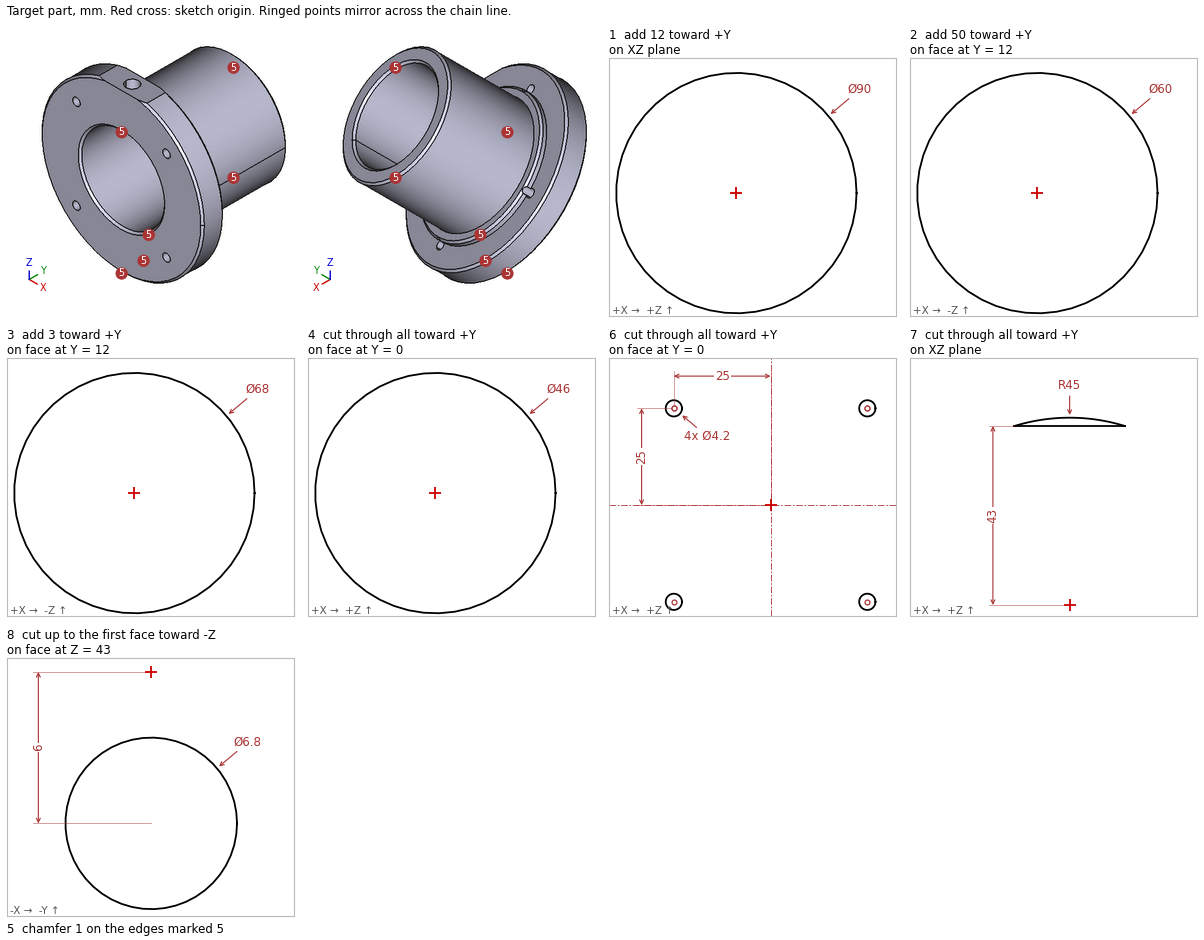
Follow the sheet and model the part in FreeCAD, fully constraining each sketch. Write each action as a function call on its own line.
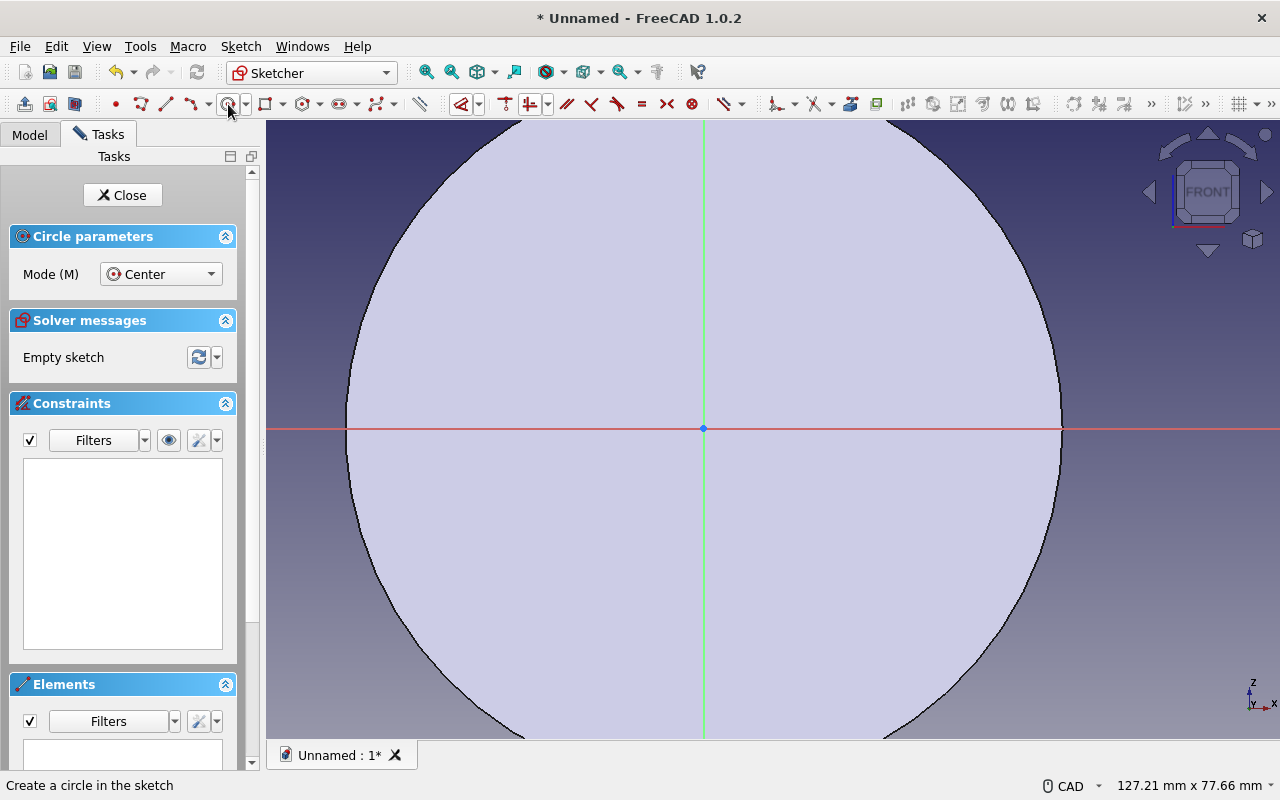
click(704, 429)
move(834, 299)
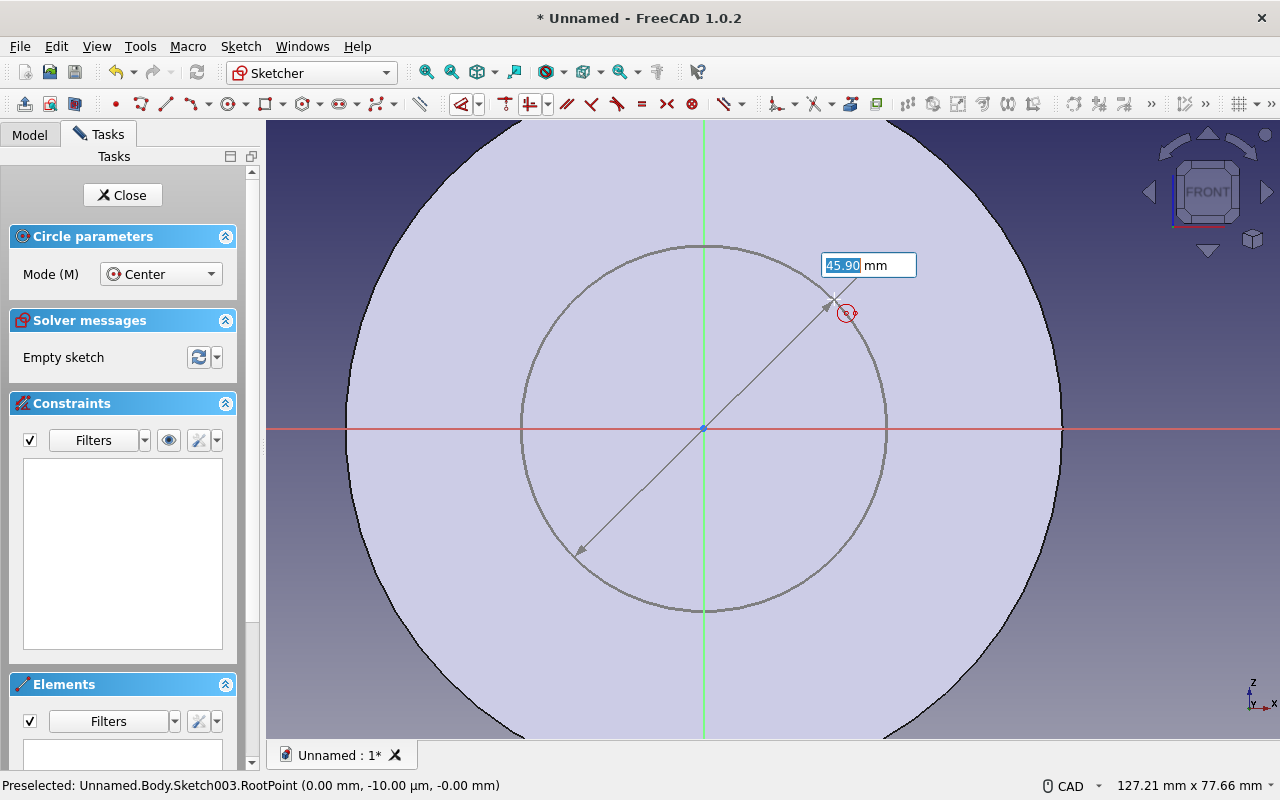
text(46)
key(Return)
key(Escape)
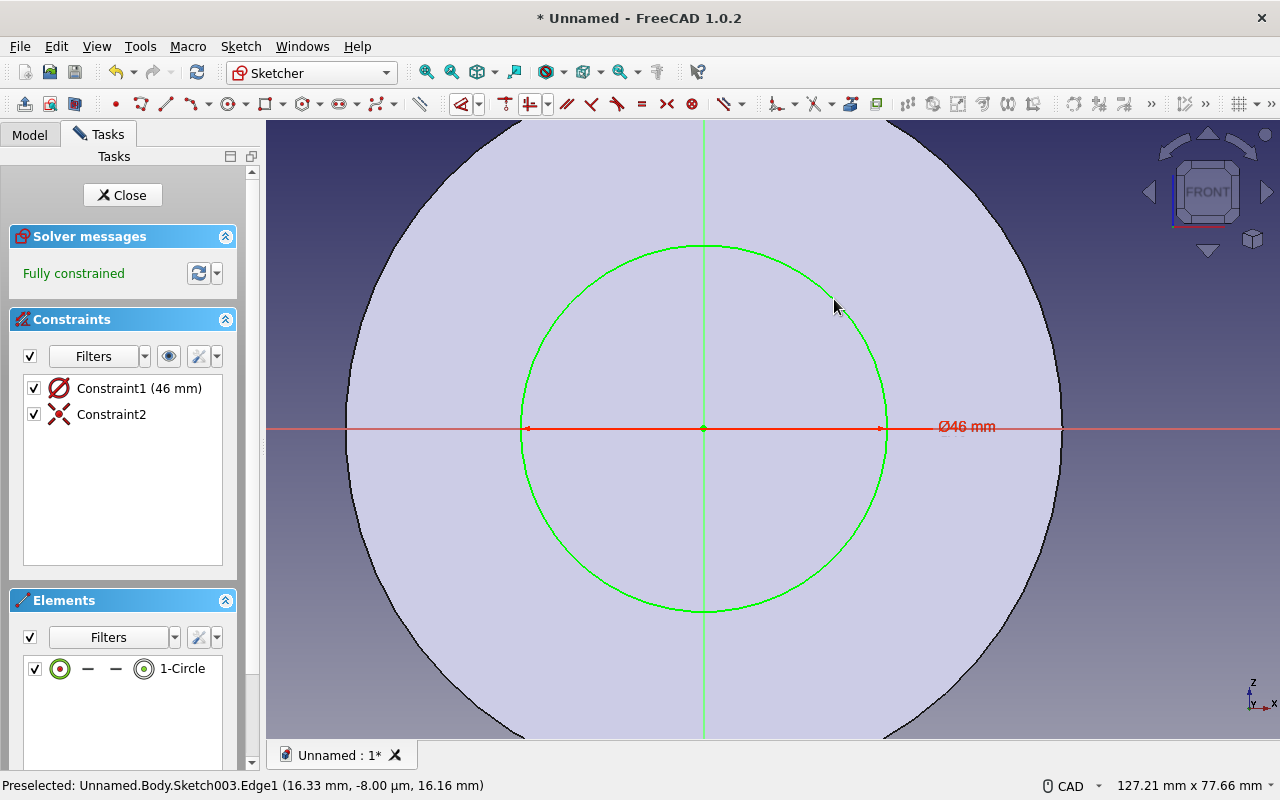
click(123, 195)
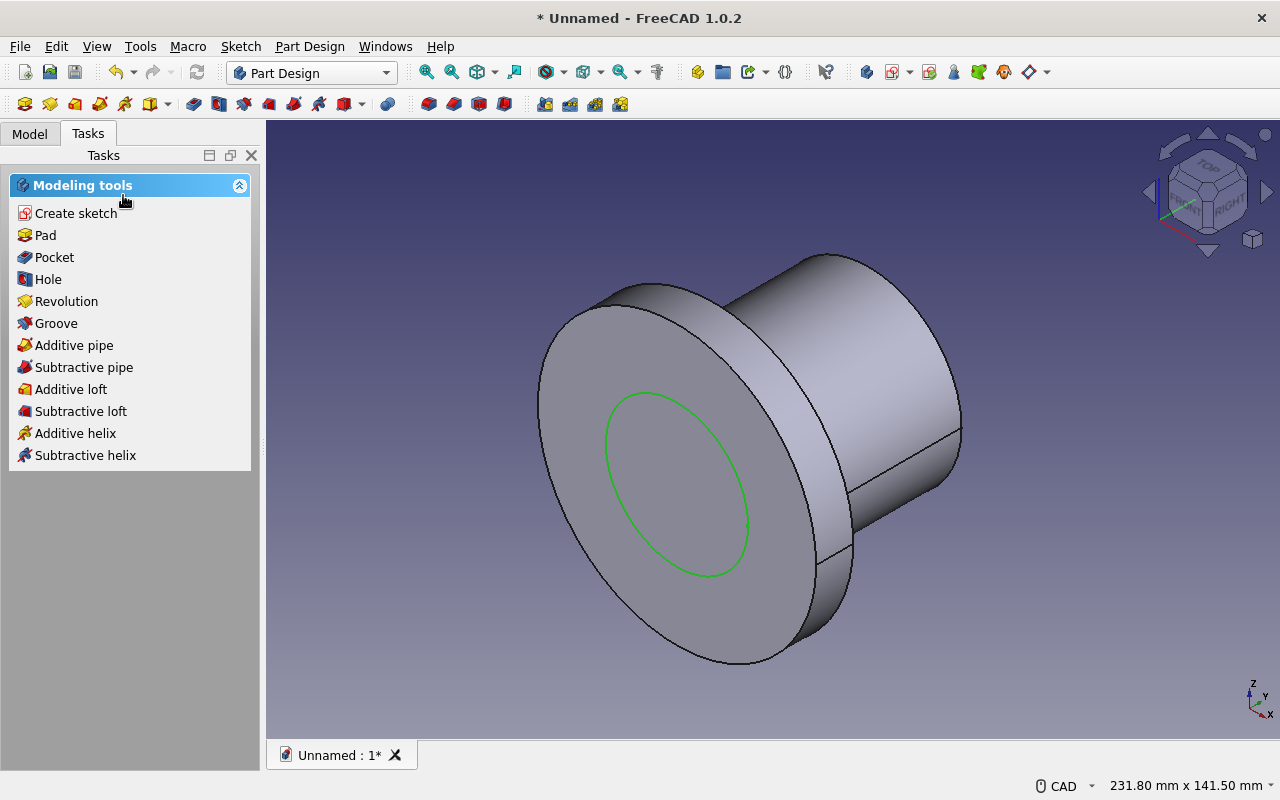
click(194, 104)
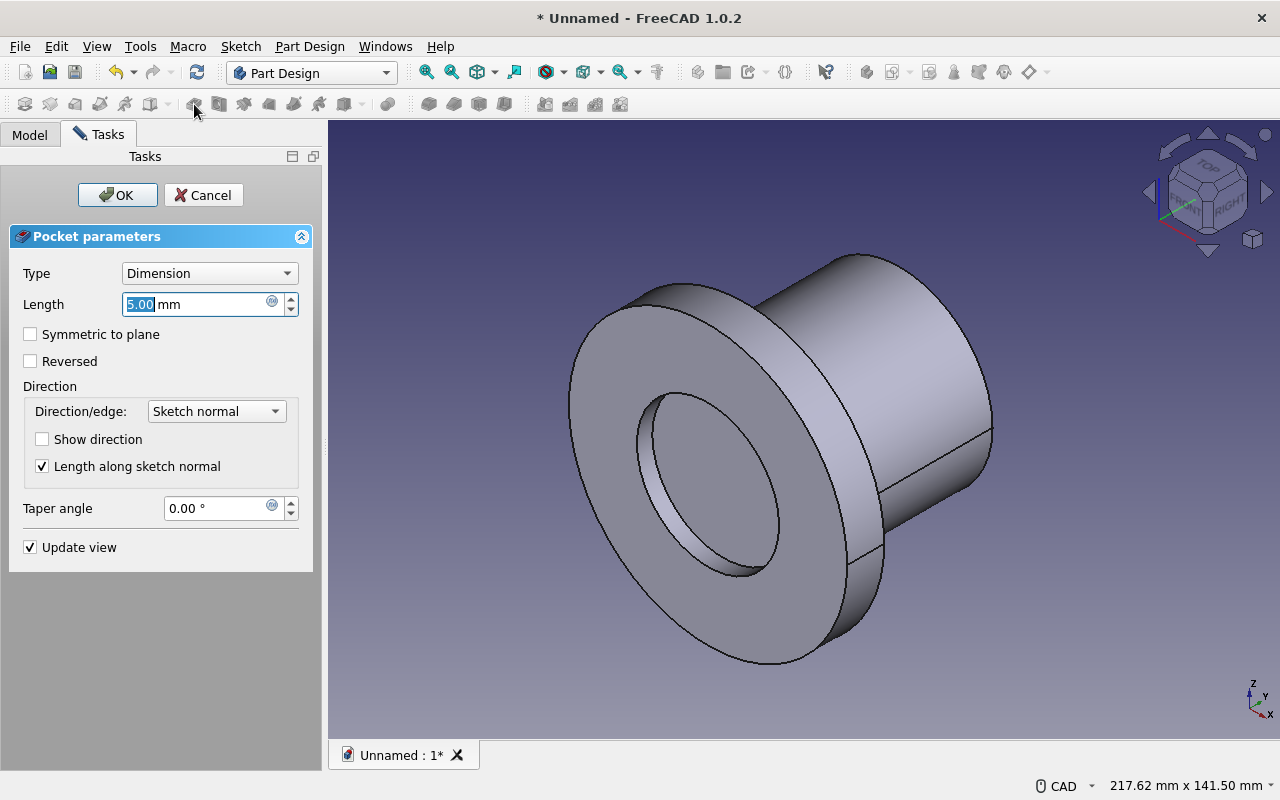
click(210, 274)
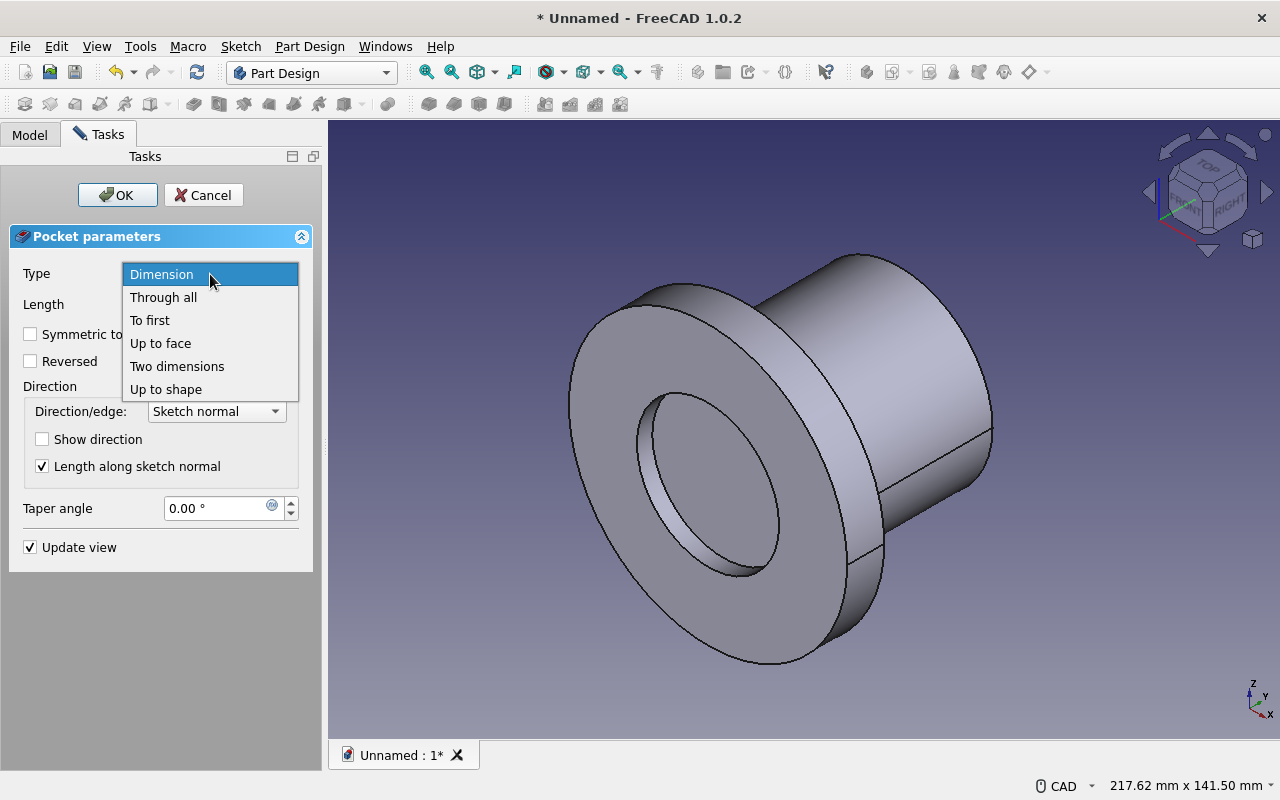
click(208, 298)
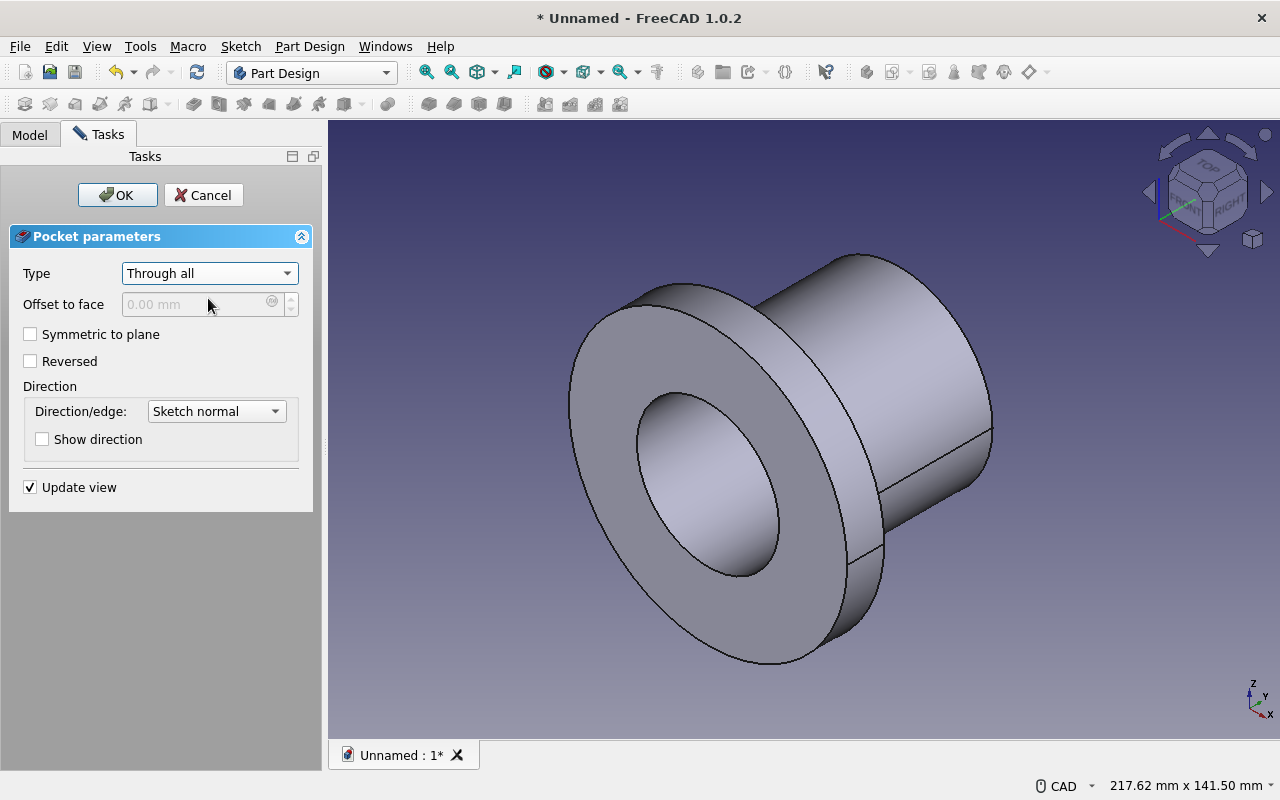
click(118, 195)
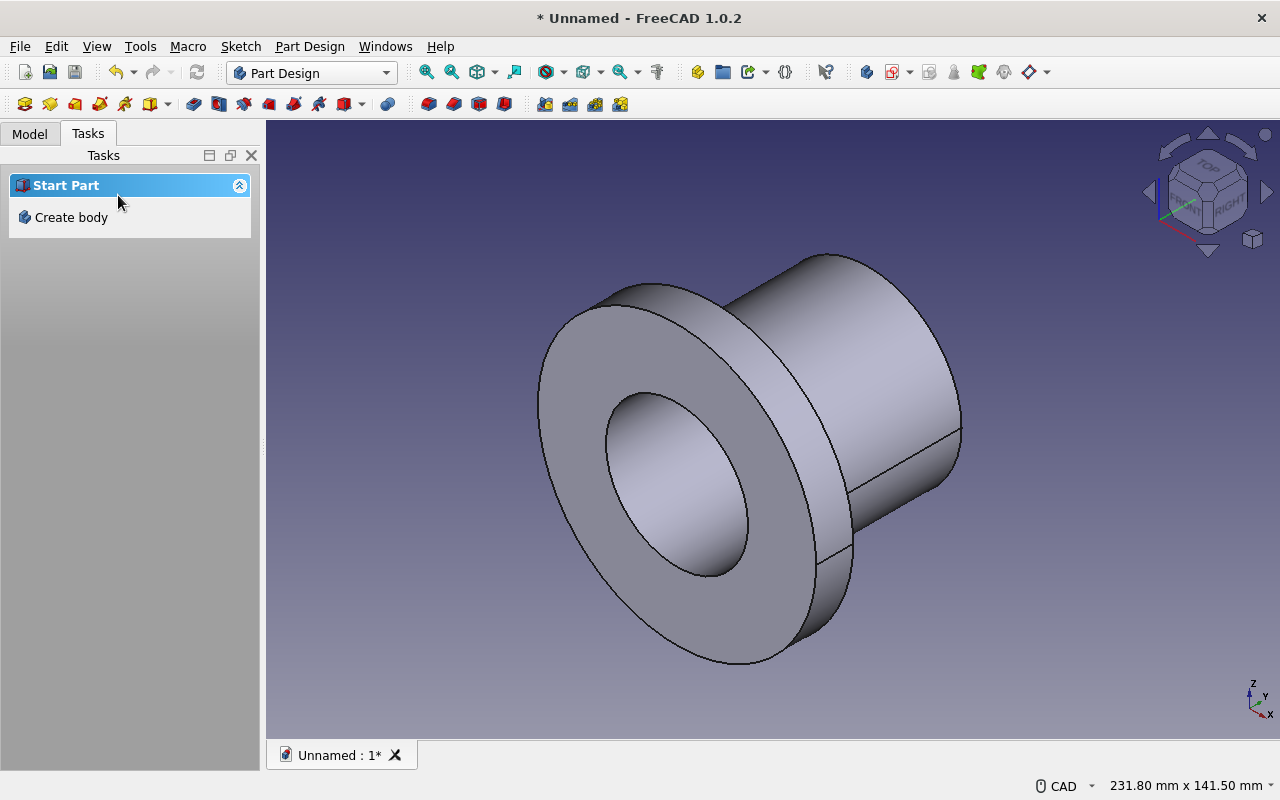
click(606, 443)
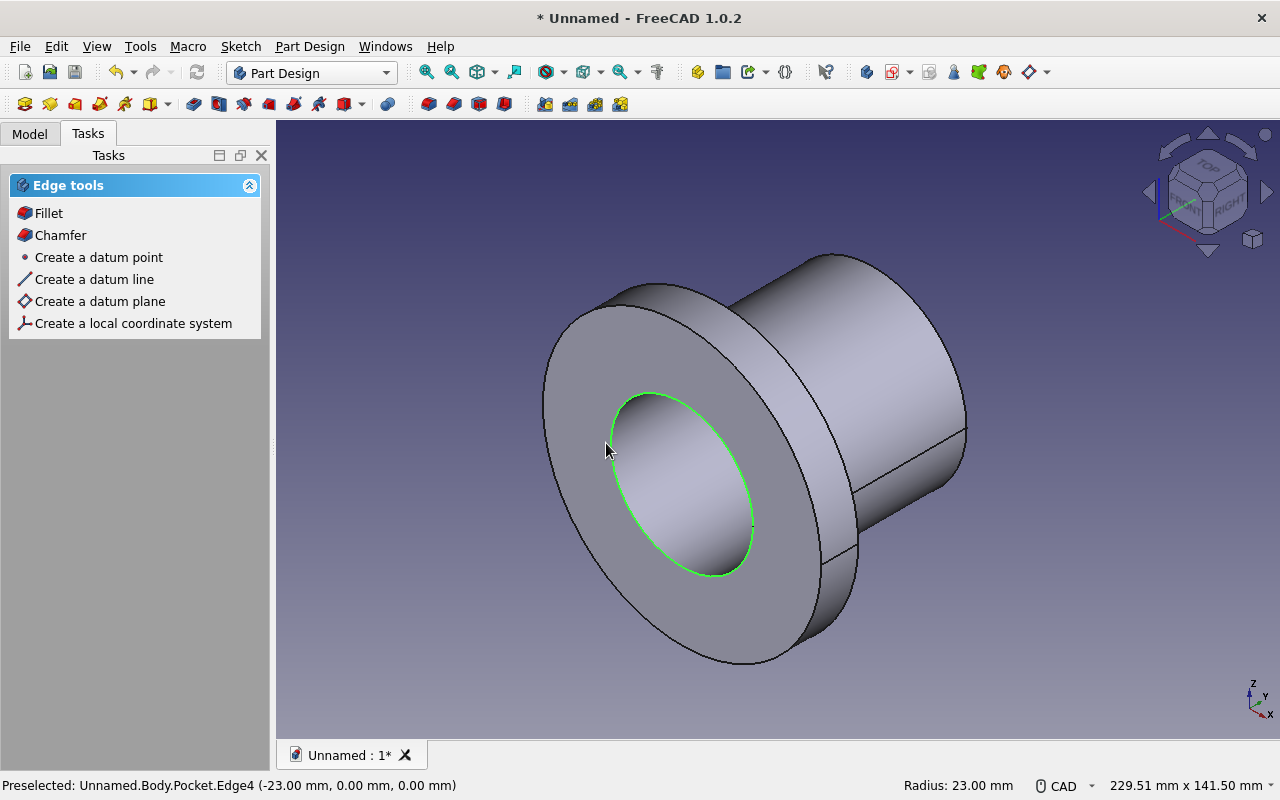
click(569, 324, ctrl)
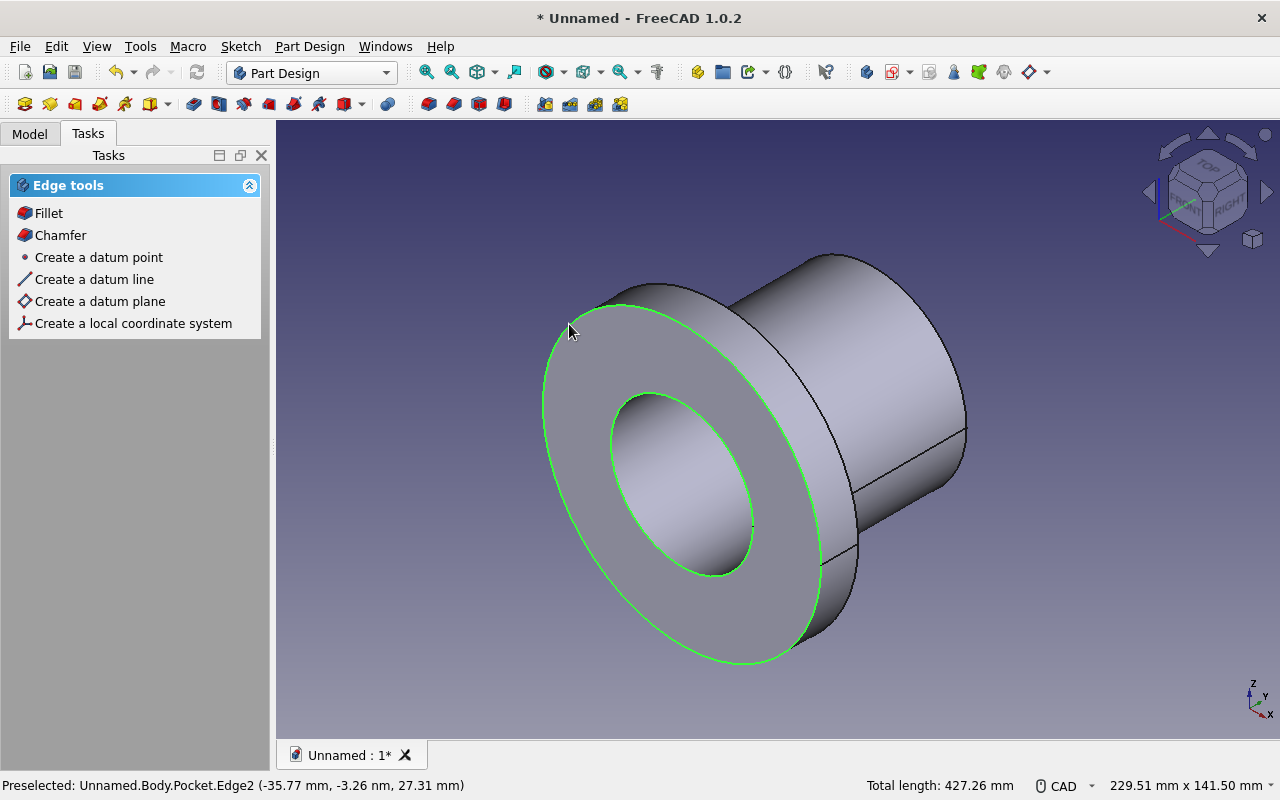
key(2)